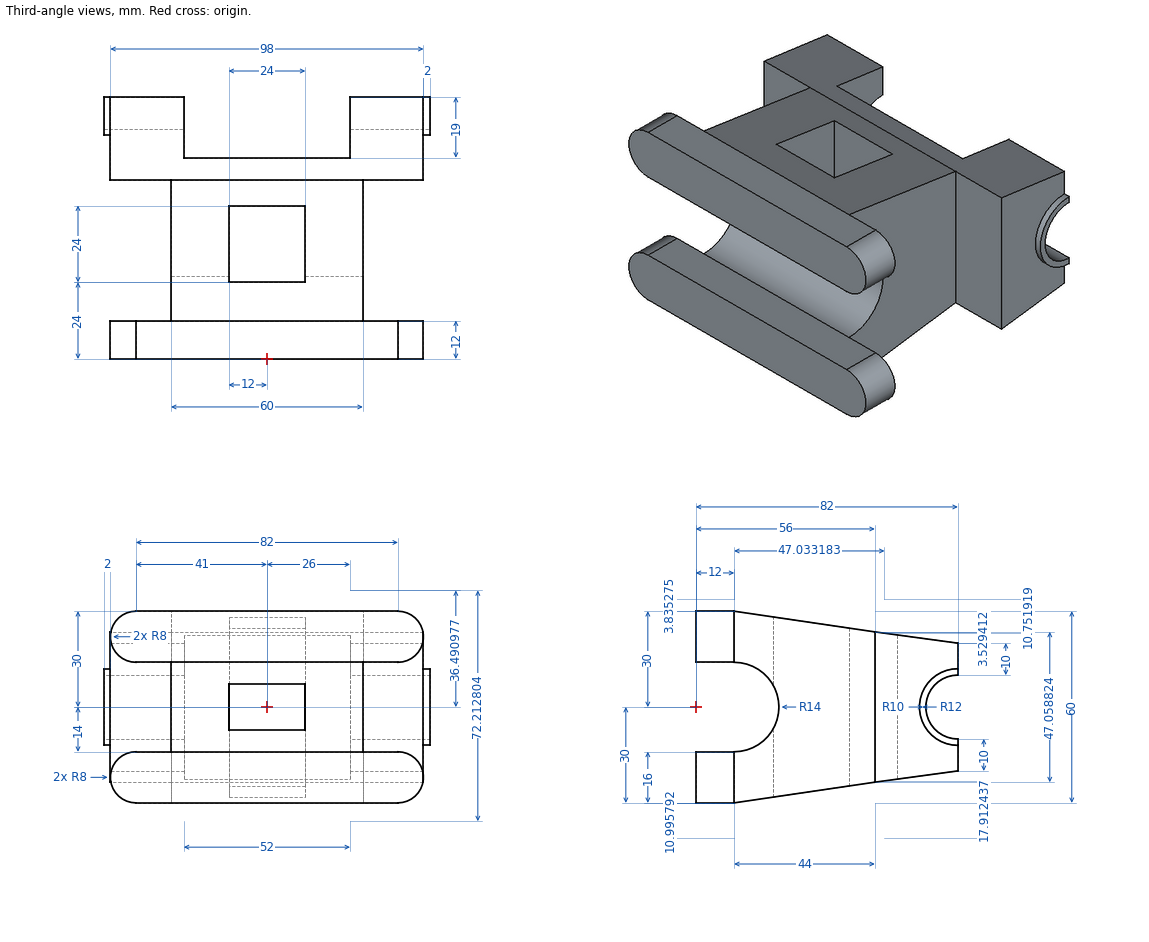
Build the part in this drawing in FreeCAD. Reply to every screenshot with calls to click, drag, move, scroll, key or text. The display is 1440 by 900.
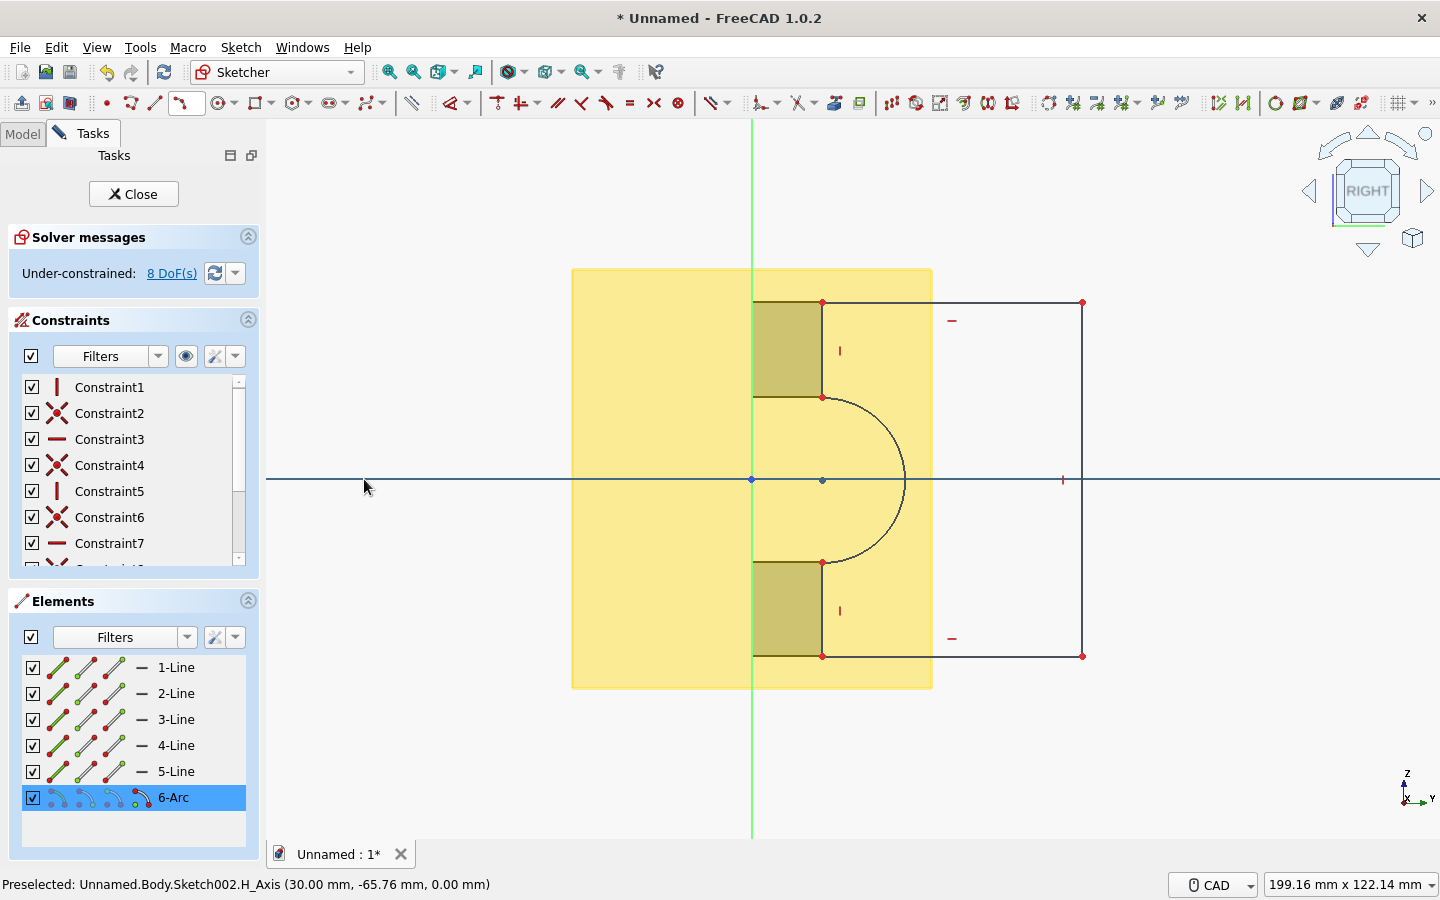
click(498, 104)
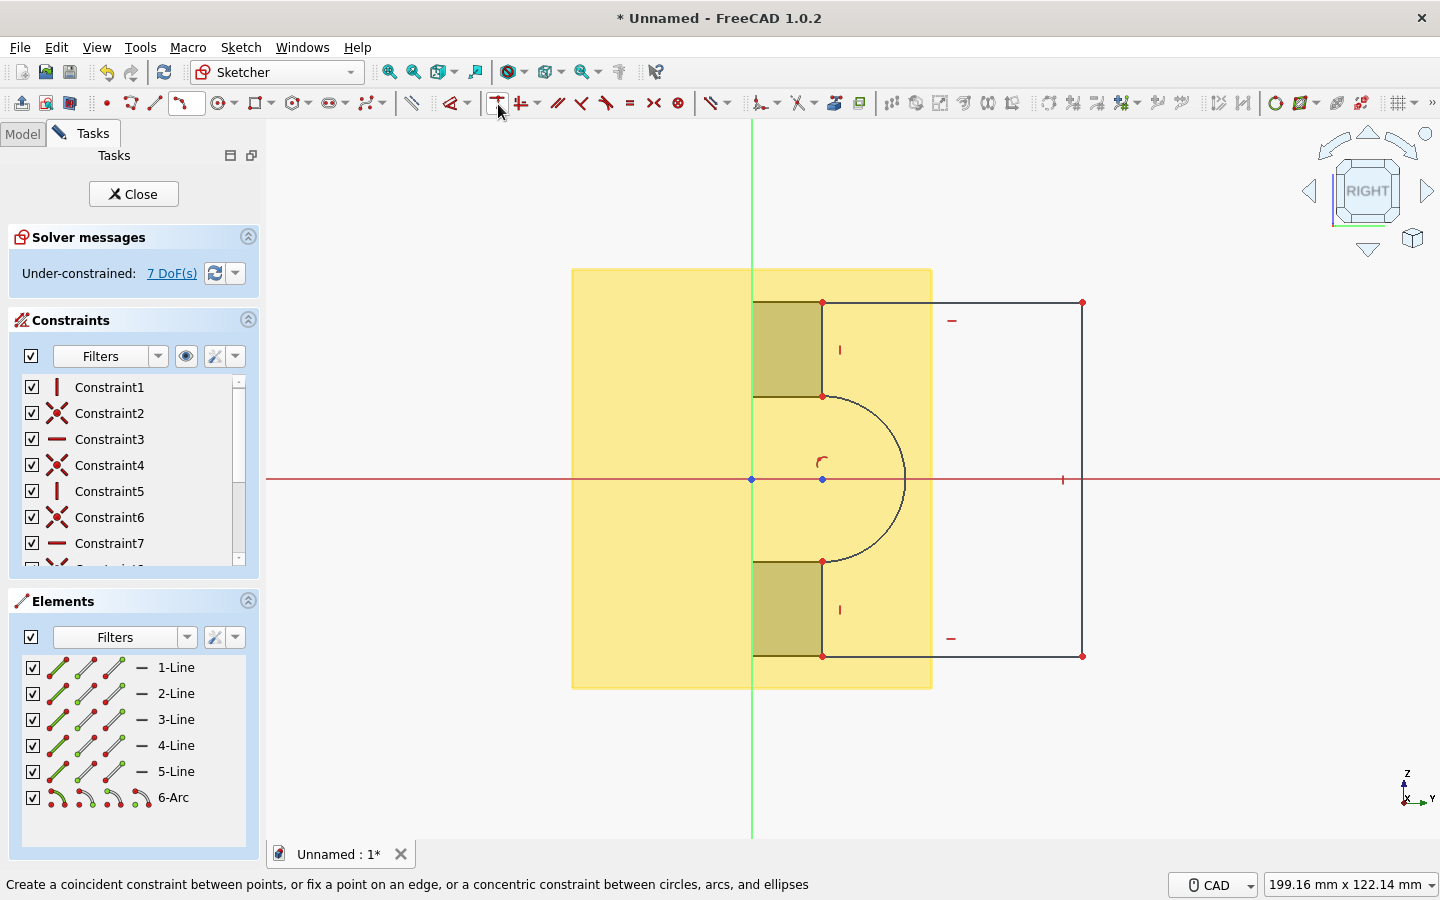
click(450, 104)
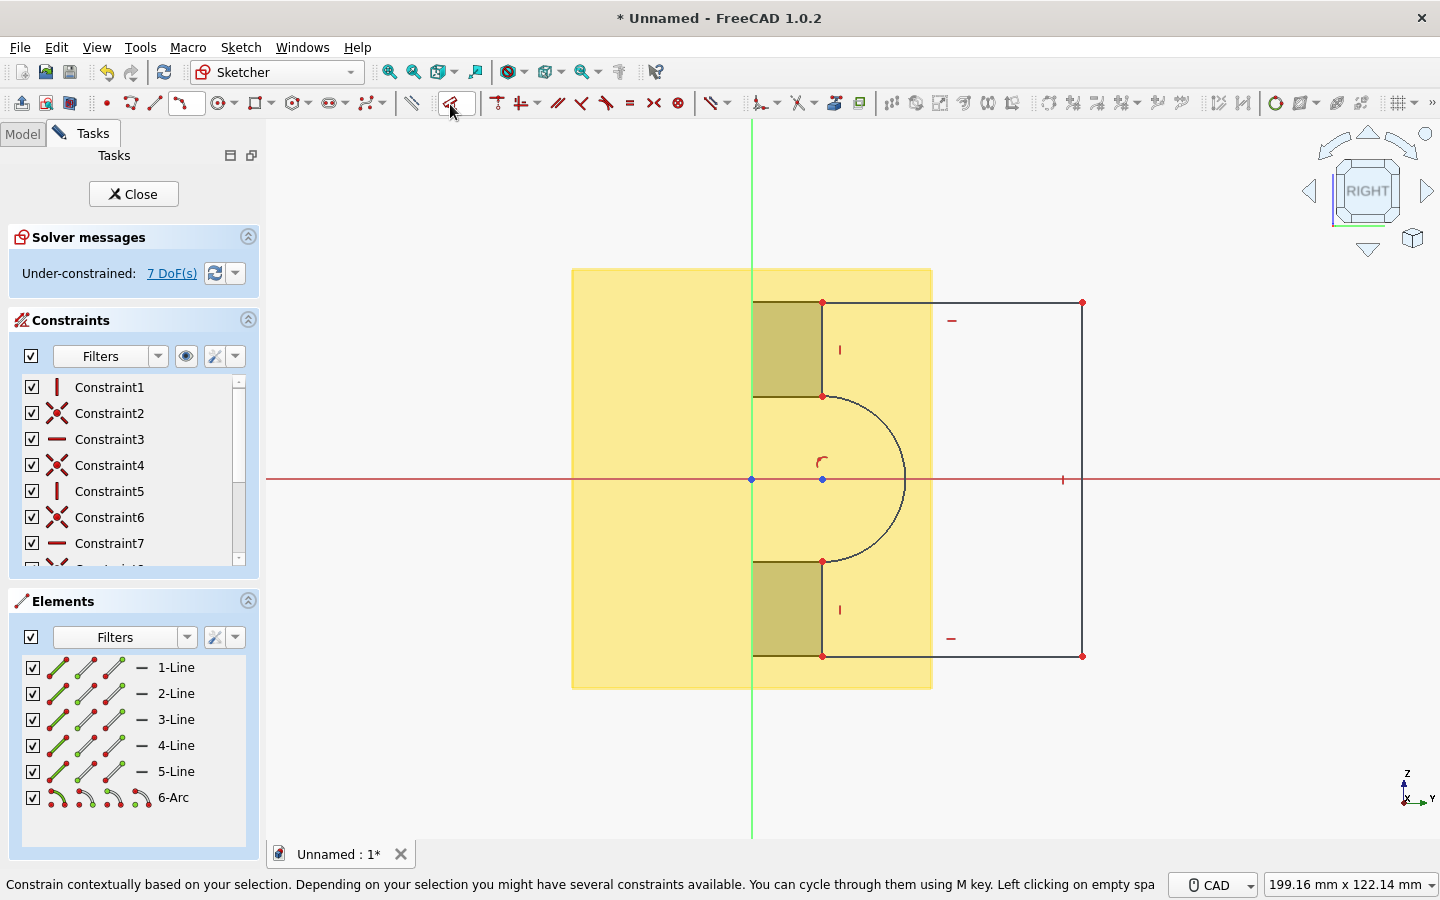
click(889, 528)
click(915, 547)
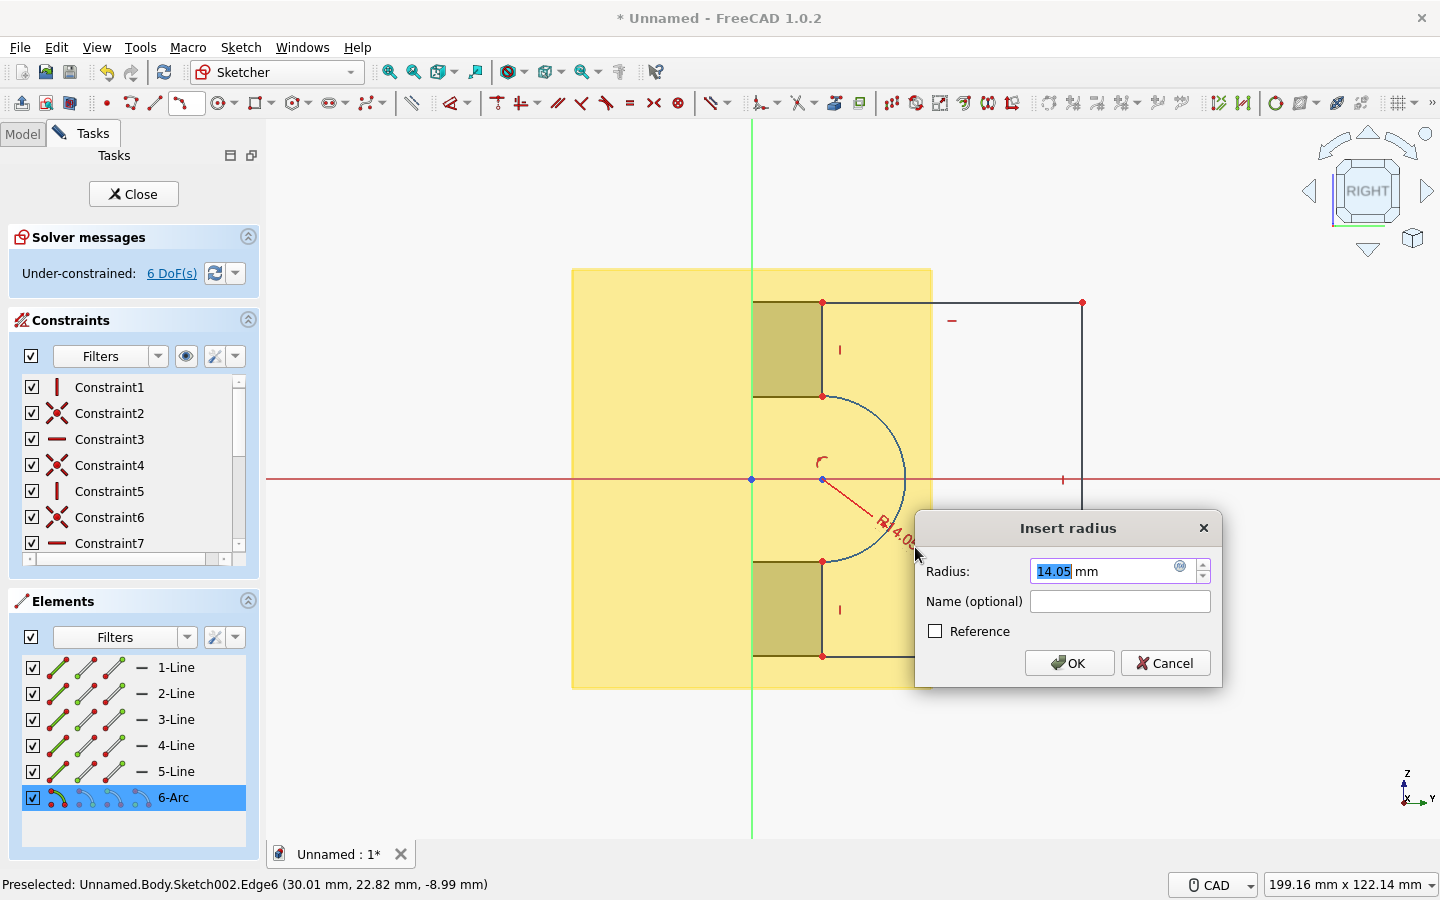
text(14)
key(Return)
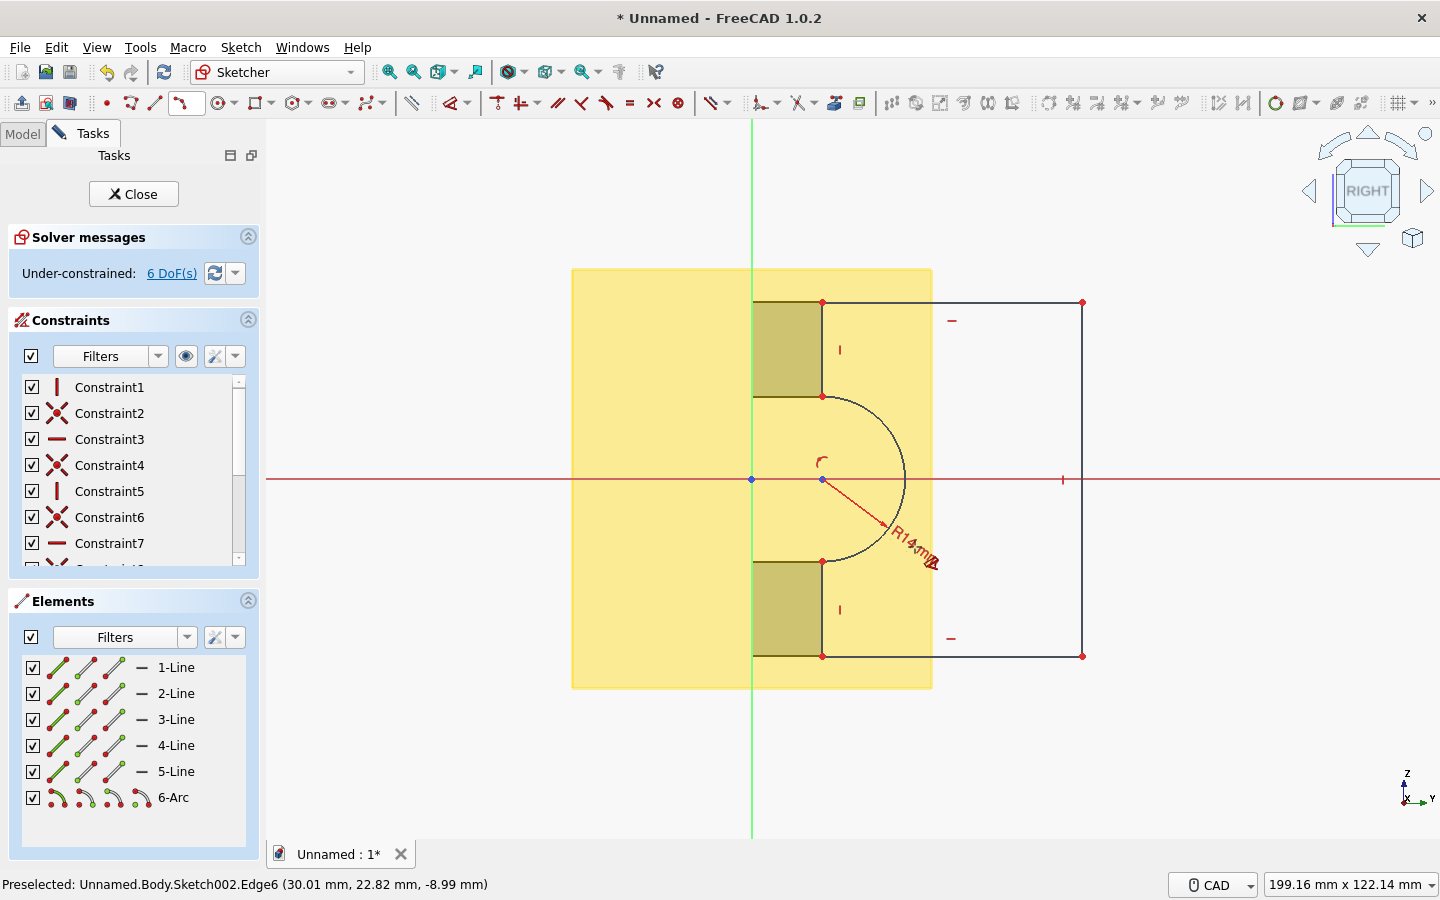
click(822, 590)
click(788, 609)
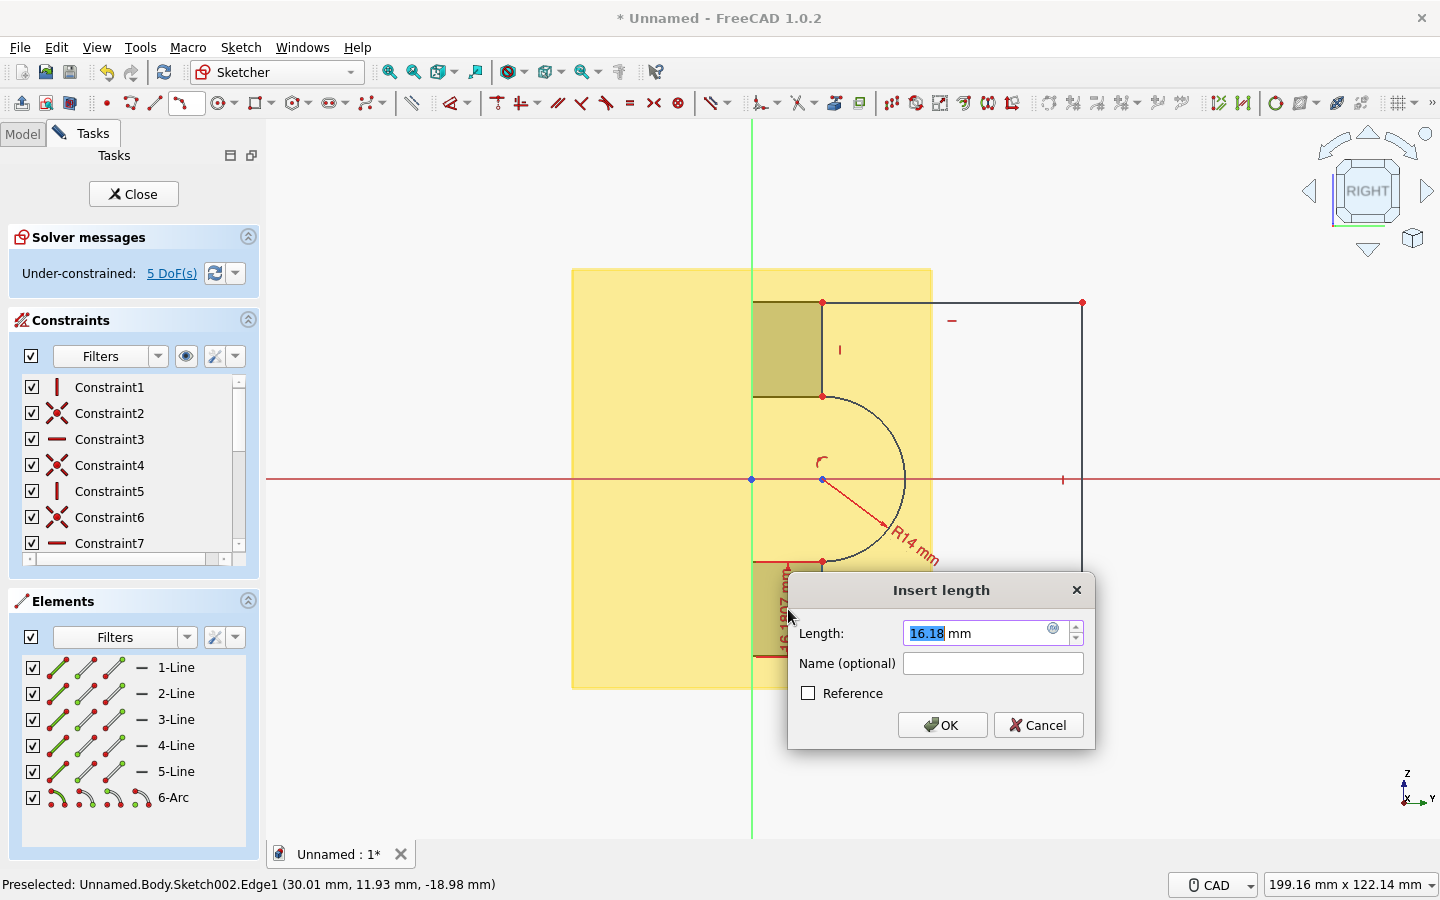
text(16)
key(Return)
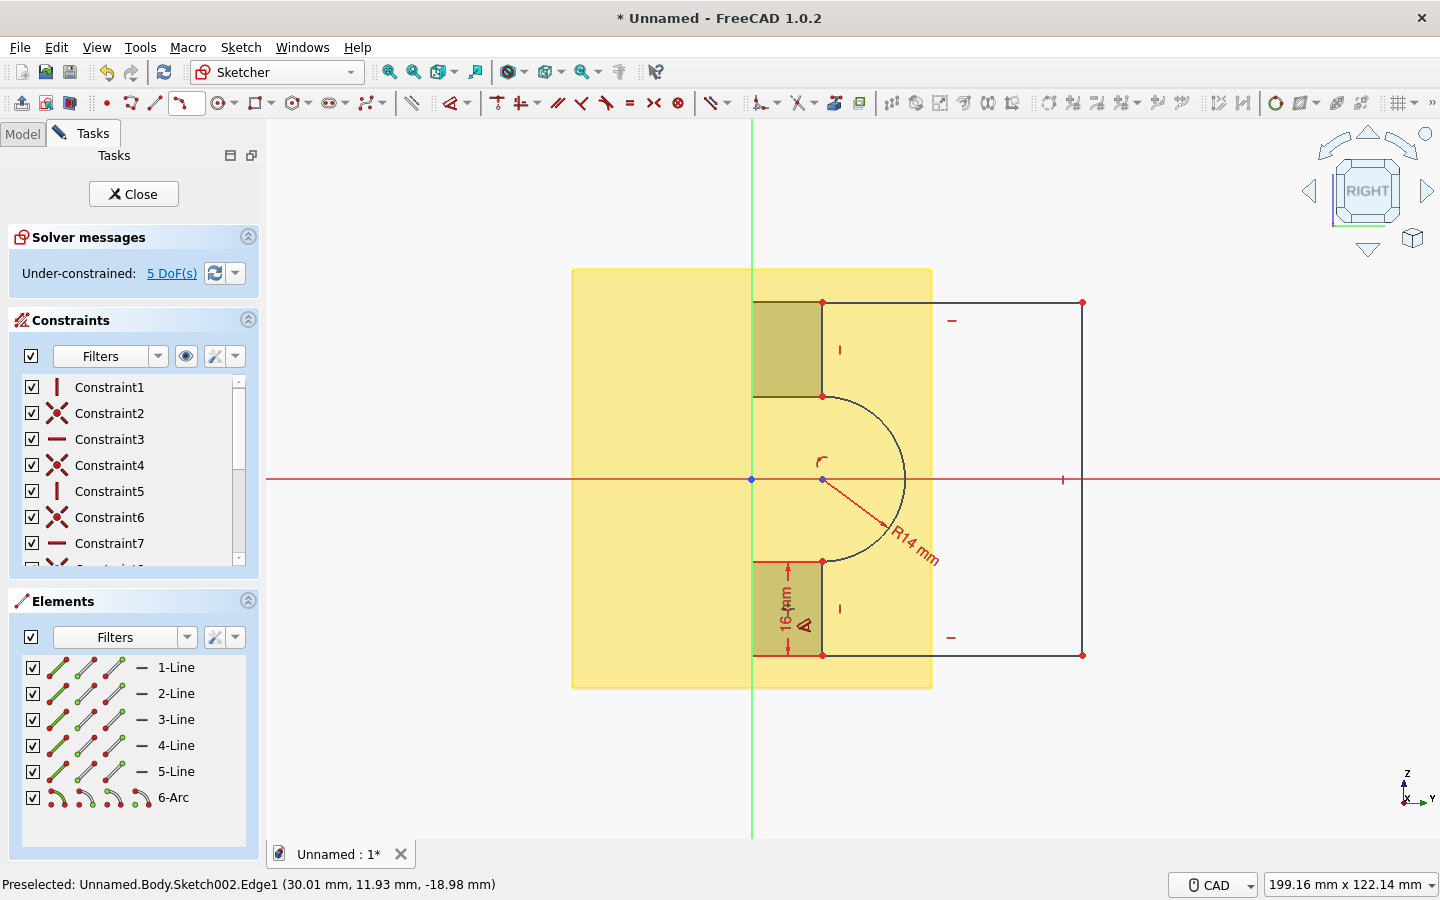
click(900, 656)
click(952, 690)